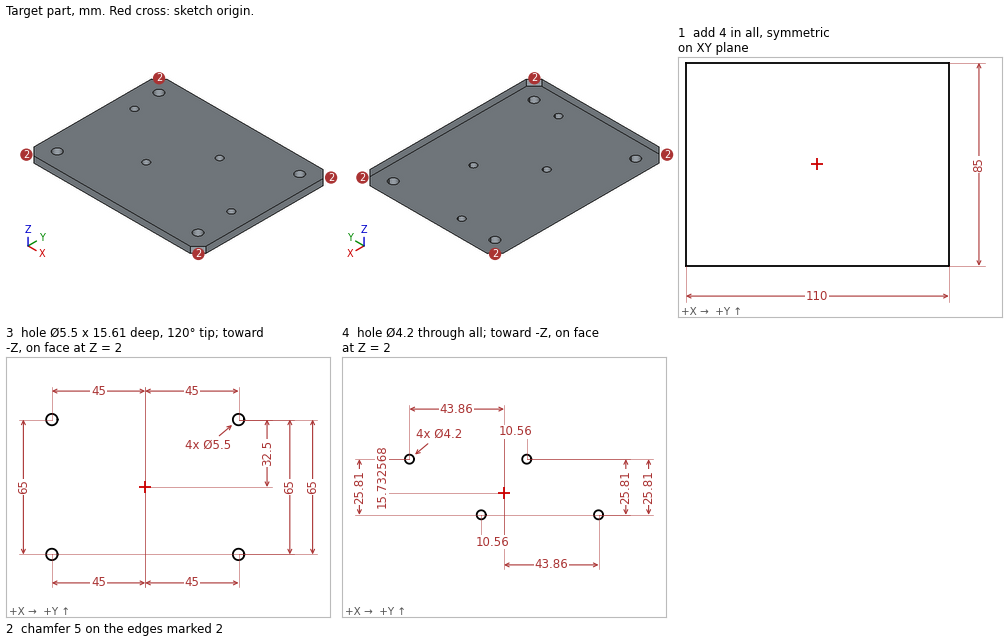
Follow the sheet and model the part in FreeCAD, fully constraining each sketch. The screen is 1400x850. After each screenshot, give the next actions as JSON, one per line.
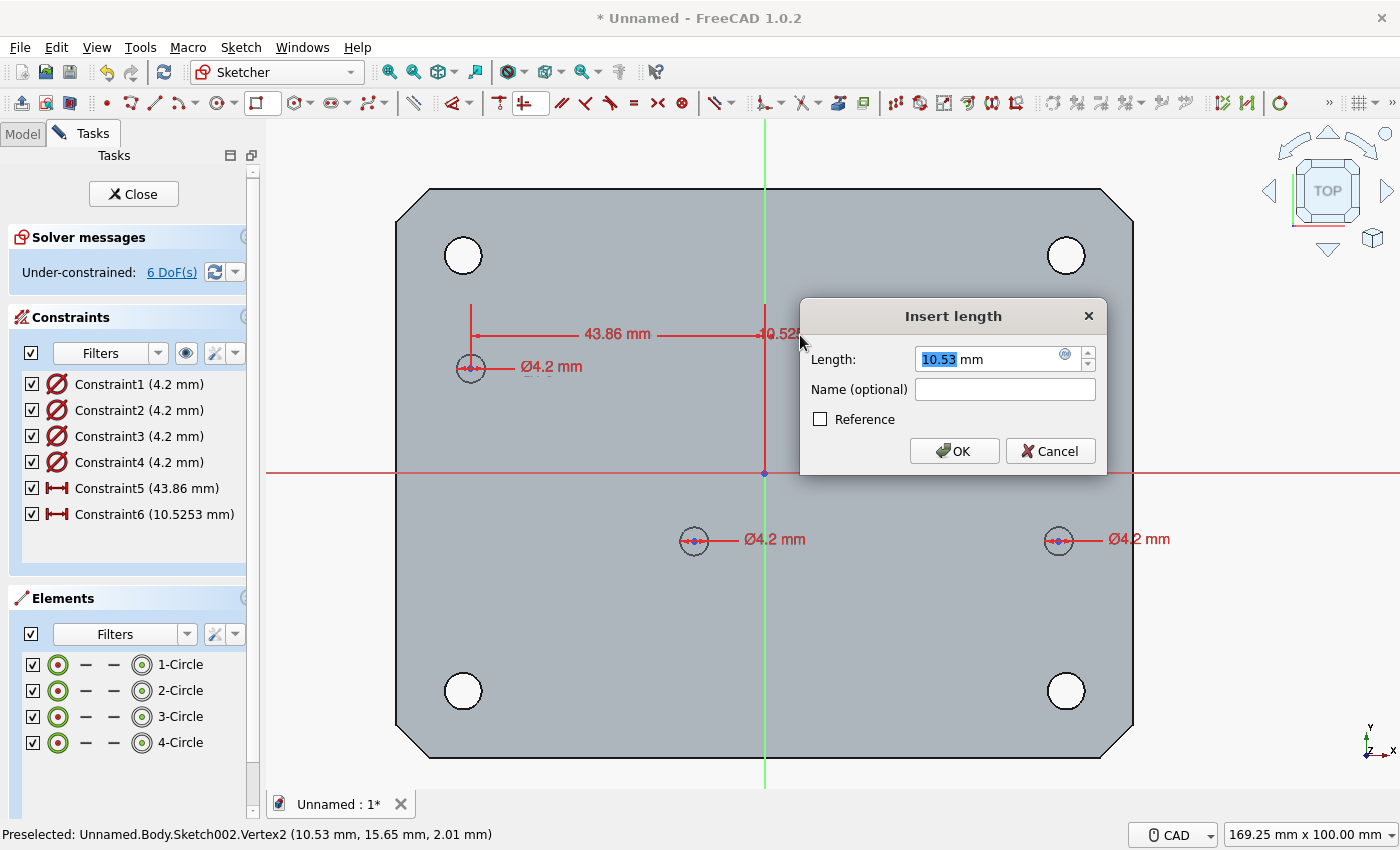
{"action": "type", "text": "10.56"}
{"action": "key", "text": "Return"}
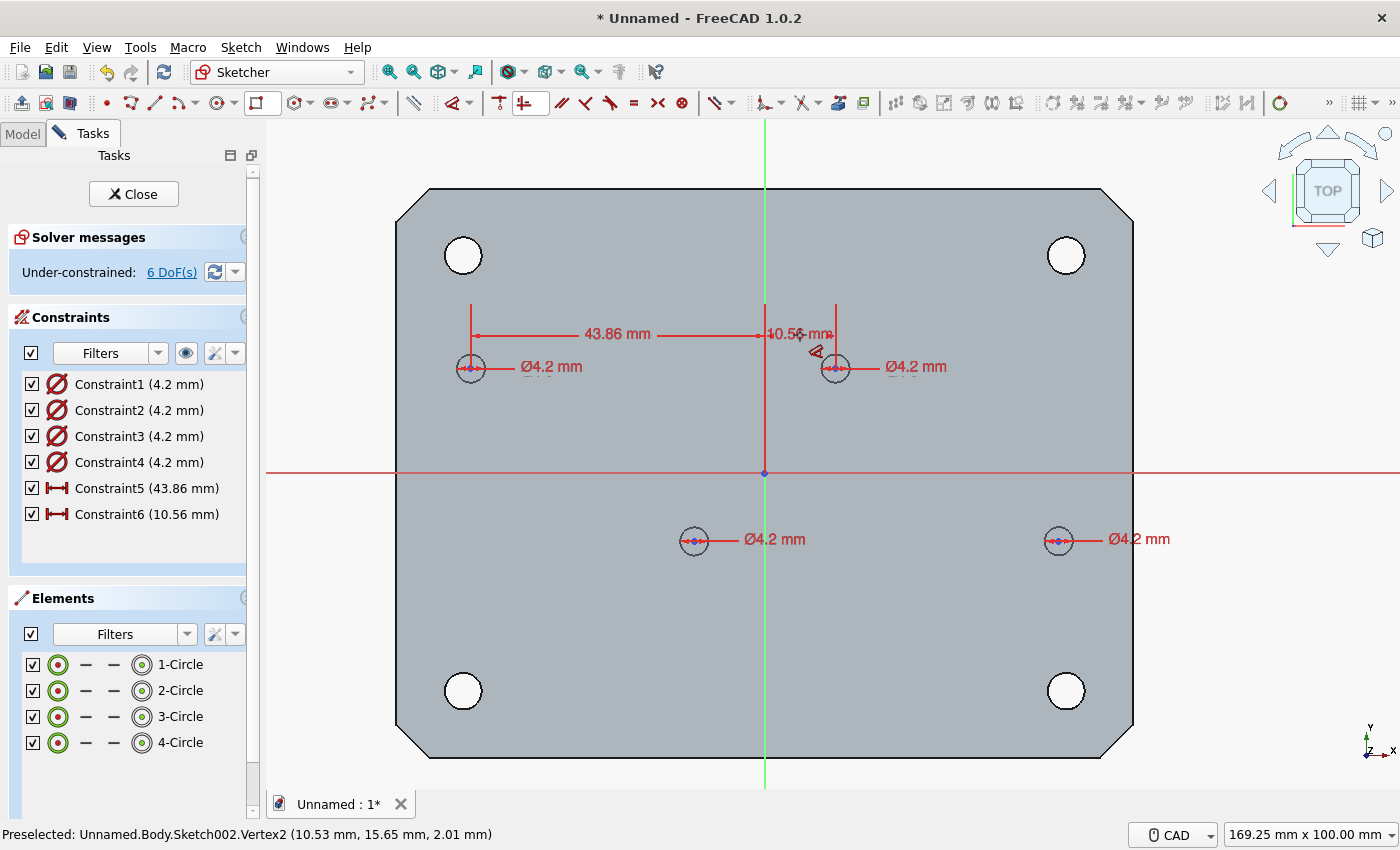
{"action": "left_click", "coordinate": [694, 541]}
{"action": "left_click", "coordinate": [730, 575]}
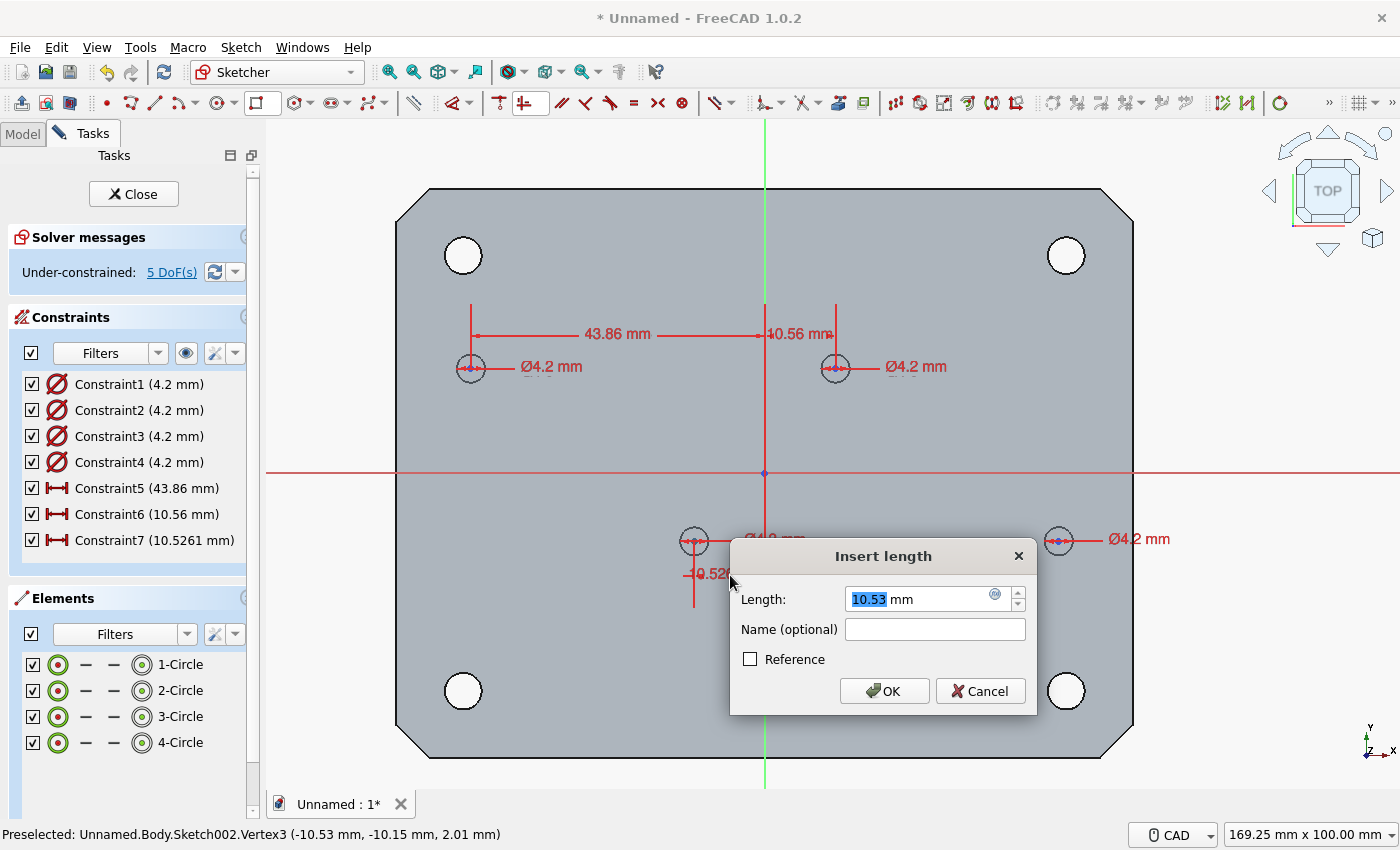
{"action": "type", "text": "10.56"}
{"action": "key", "text": "Return"}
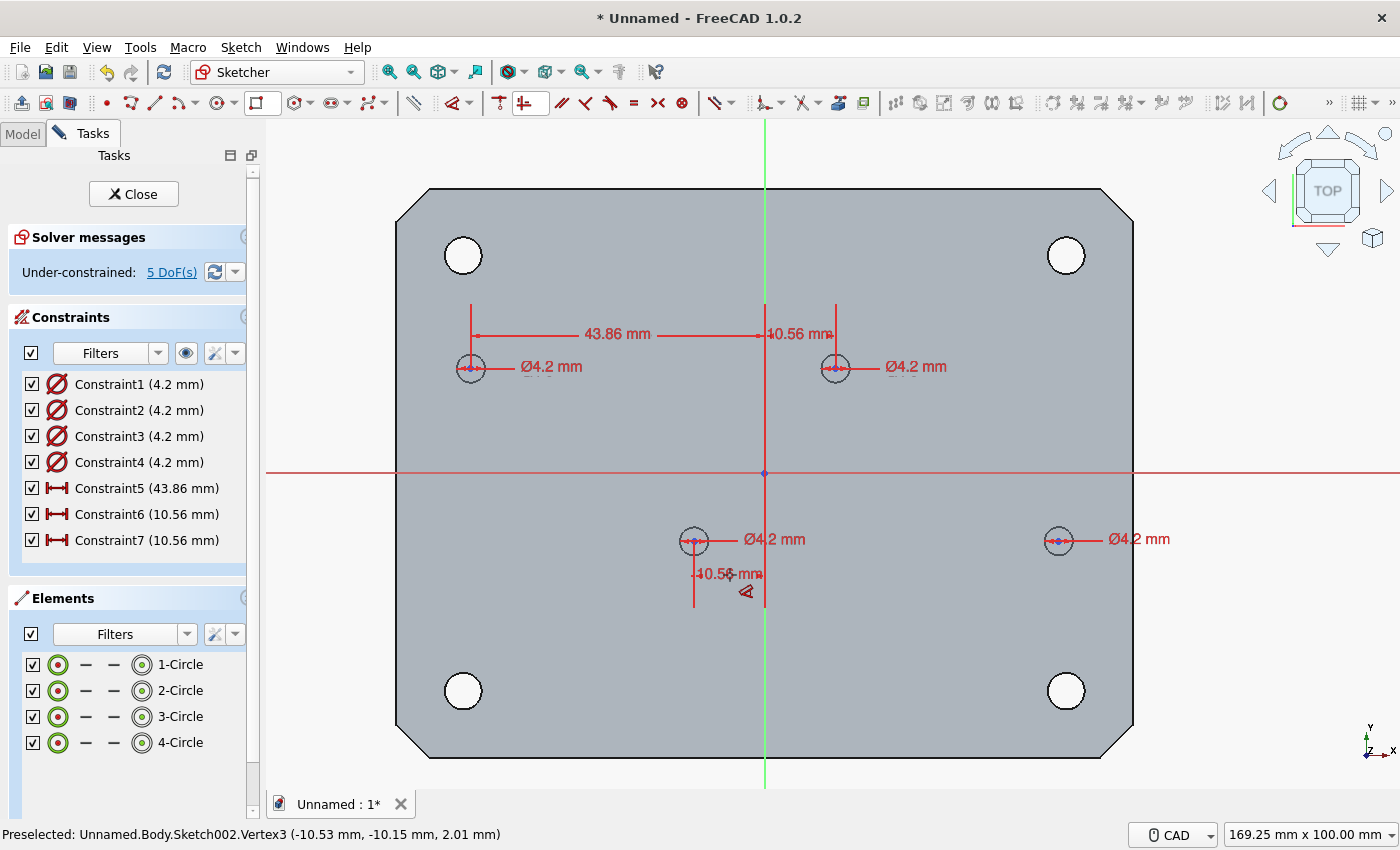
{"action": "left_click", "coordinate": [1059, 541]}
{"action": "left_click", "coordinate": [912, 575]}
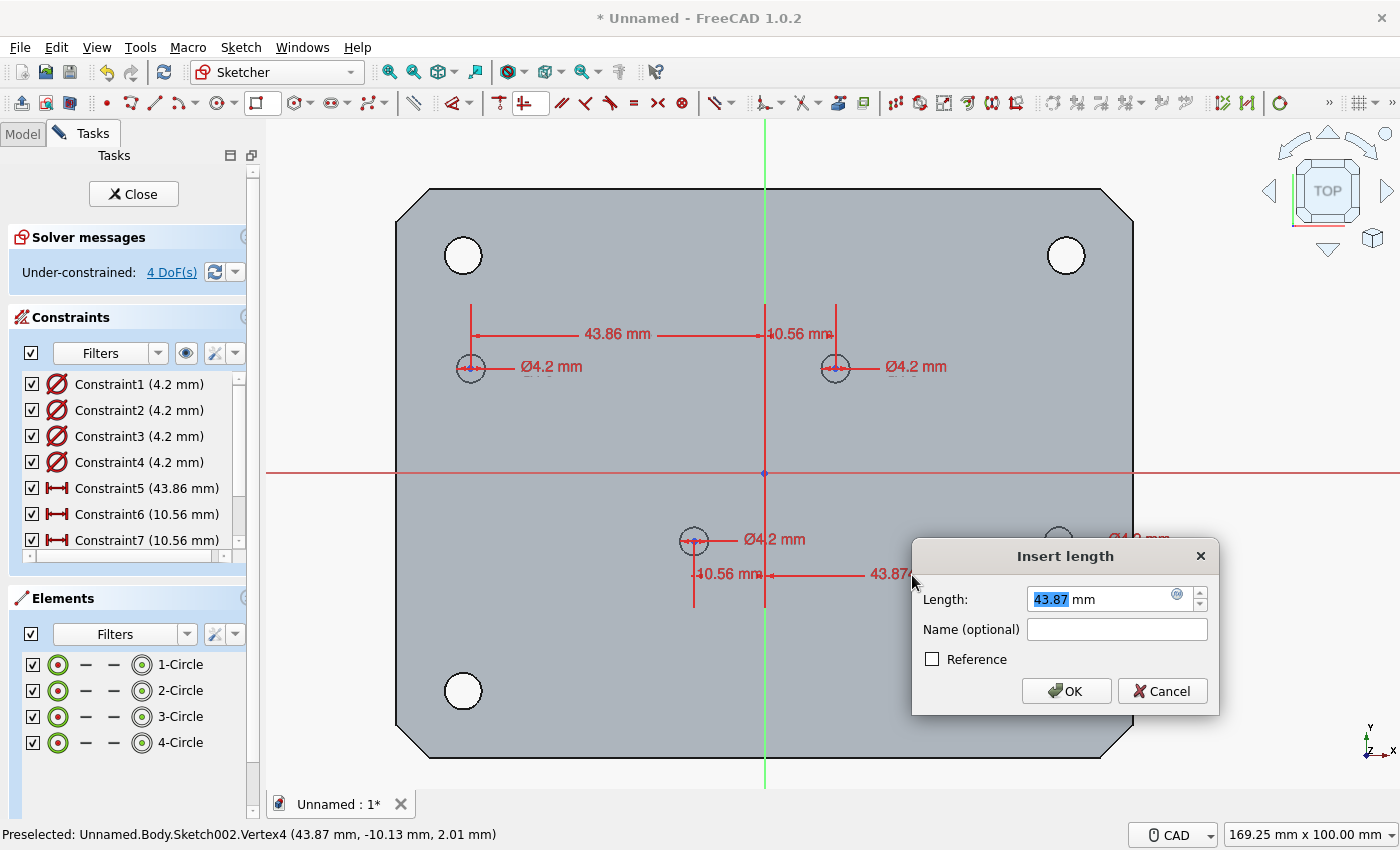
{"action": "type", "text": "43.86"}
{"action": "key", "text": "Return"}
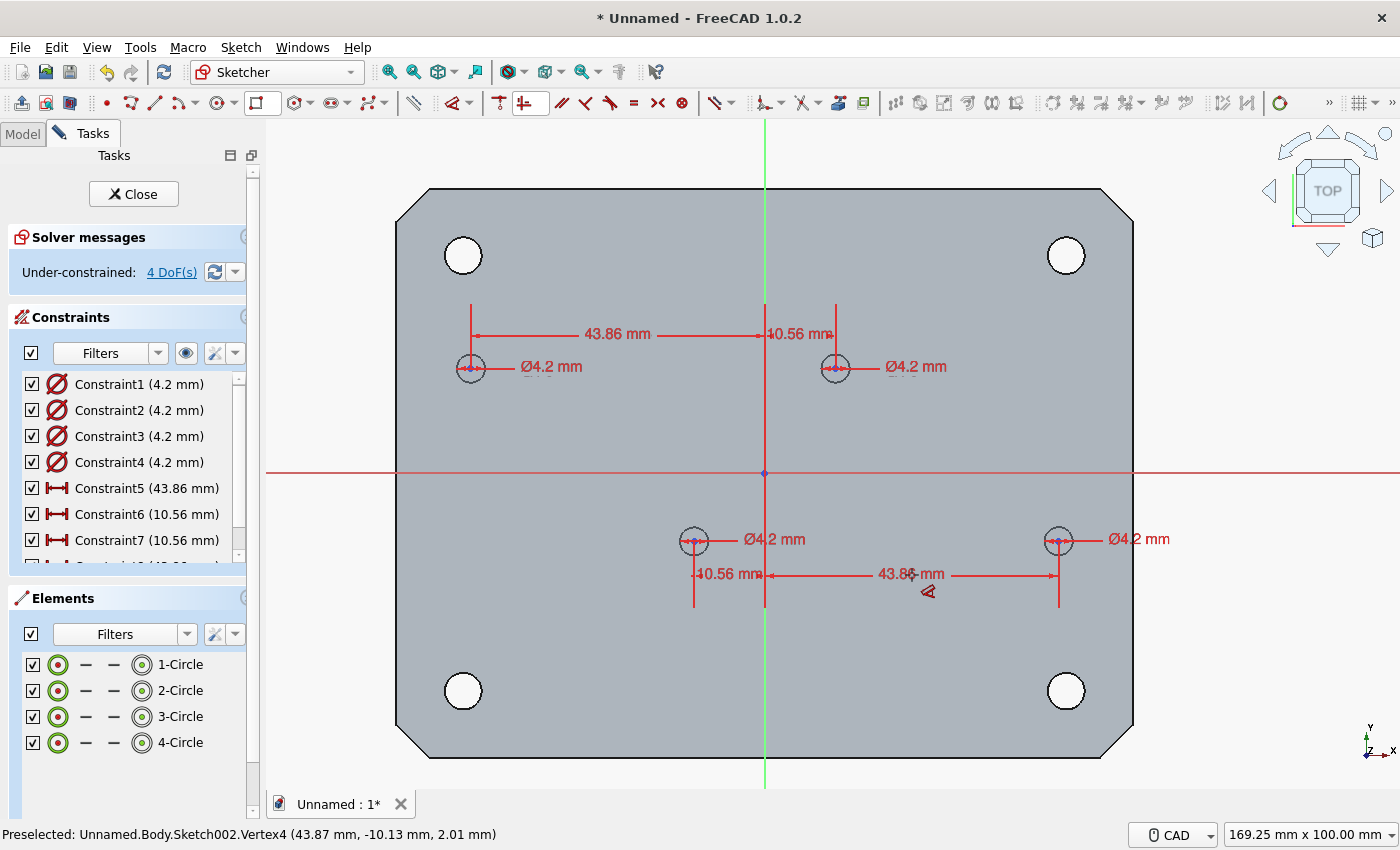
{"action": "left_click", "coordinate": [836, 369]}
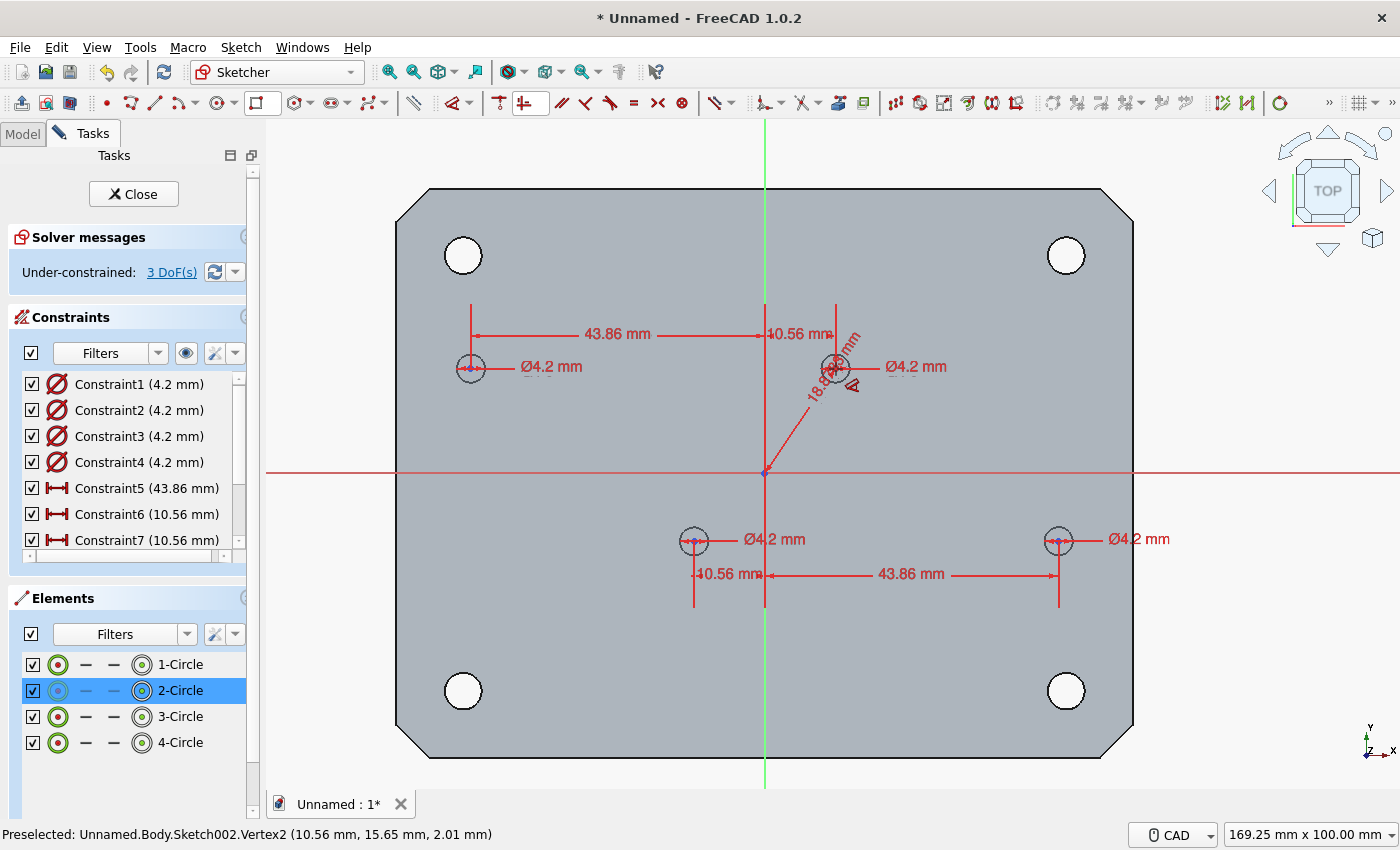
{"action": "left_click", "coordinate": [694, 541]}
{"action": "left_click", "coordinate": [870, 455]}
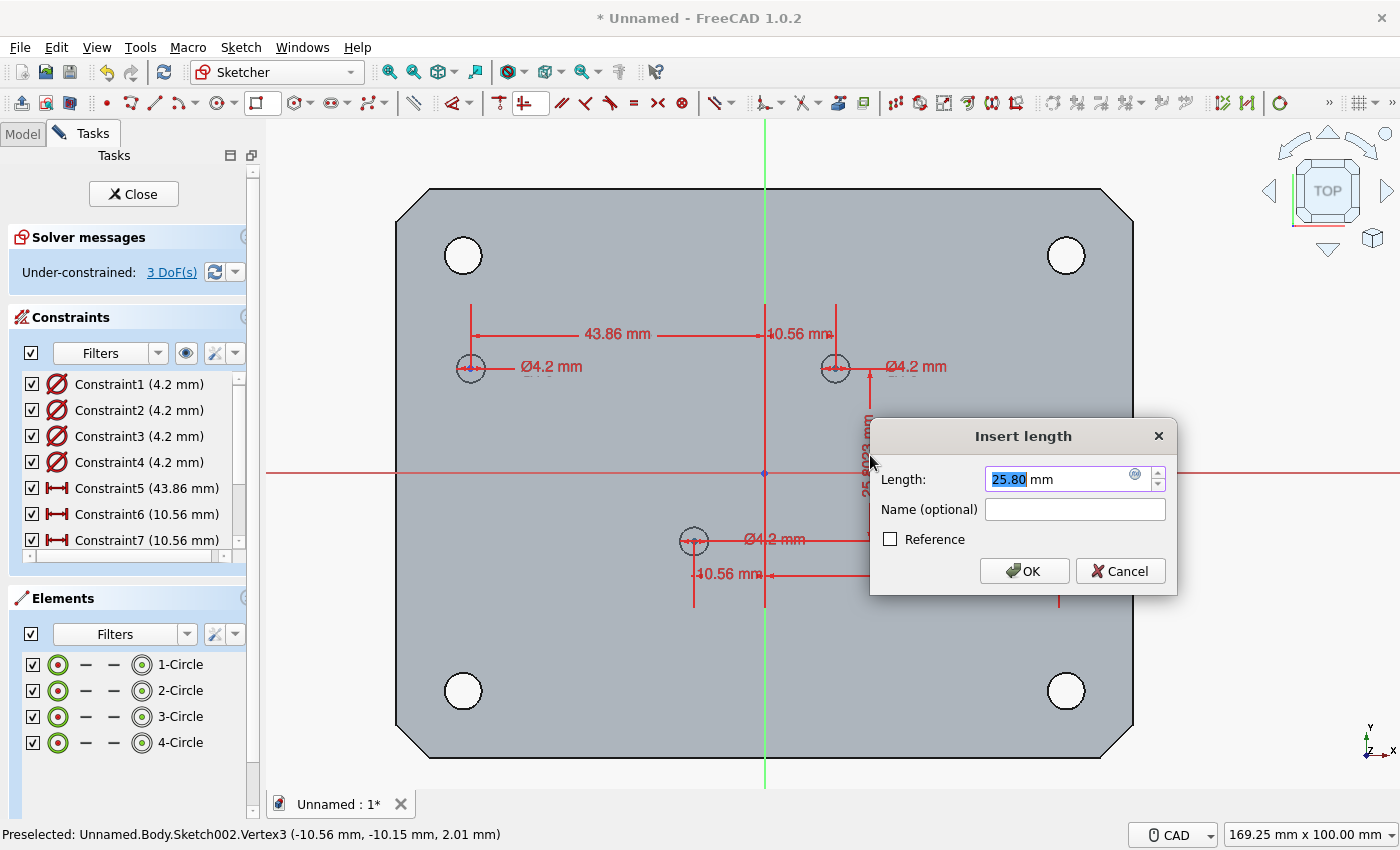
{"action": "type", "text": "25.81"}
{"action": "key", "text": "Return"}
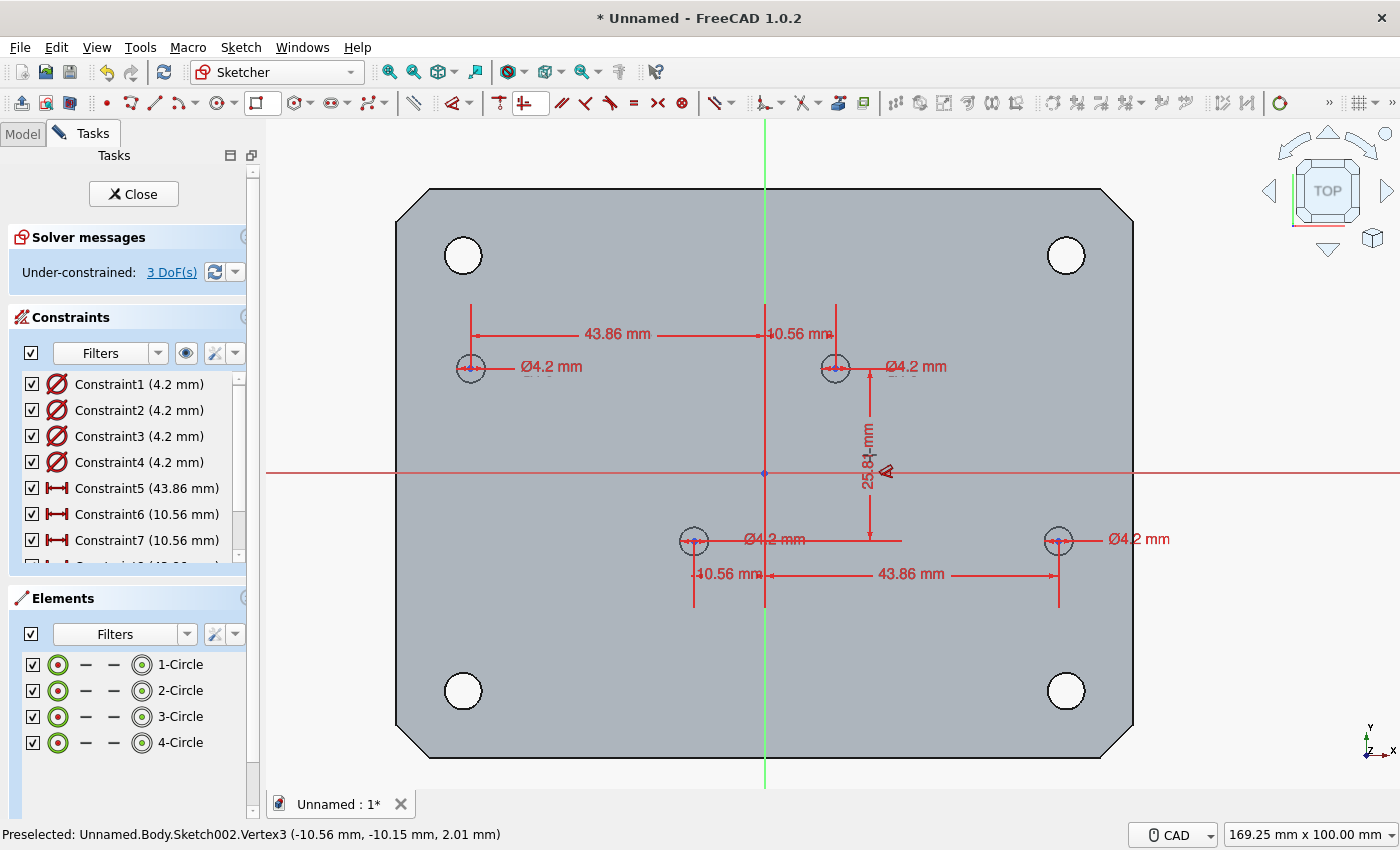
{"action": "left_click", "coordinate": [471, 369]}